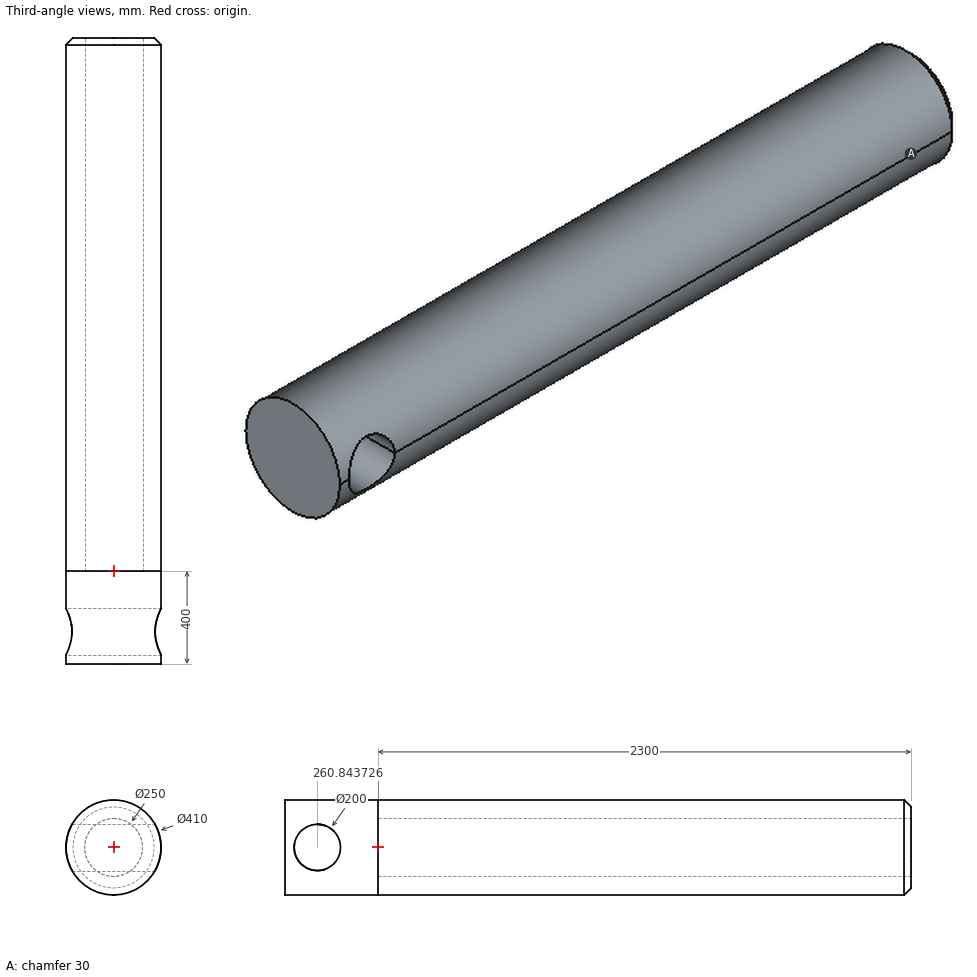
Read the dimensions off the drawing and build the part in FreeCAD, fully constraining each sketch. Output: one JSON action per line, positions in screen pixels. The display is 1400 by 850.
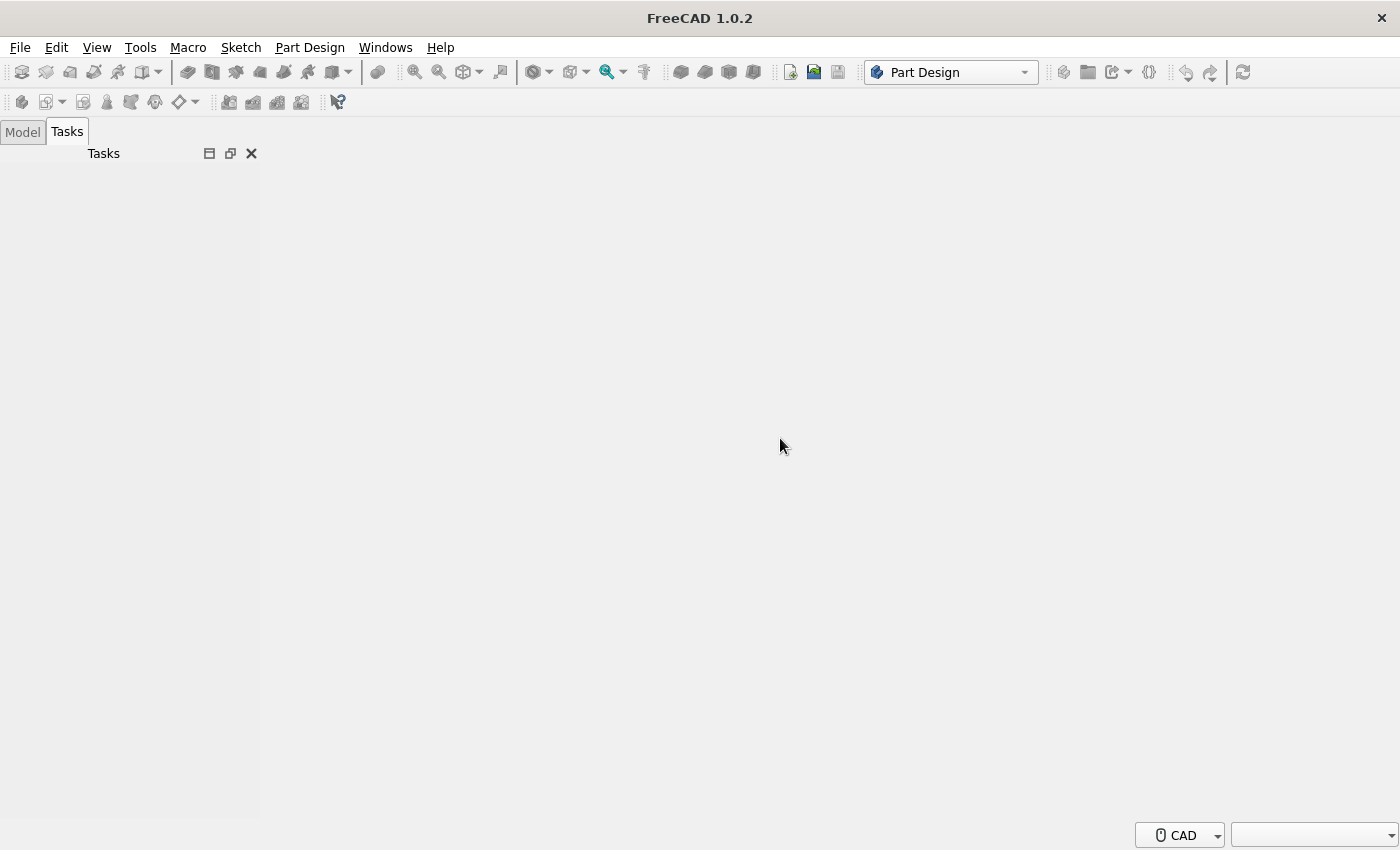
{"action": "left_click", "coordinate": [790, 72]}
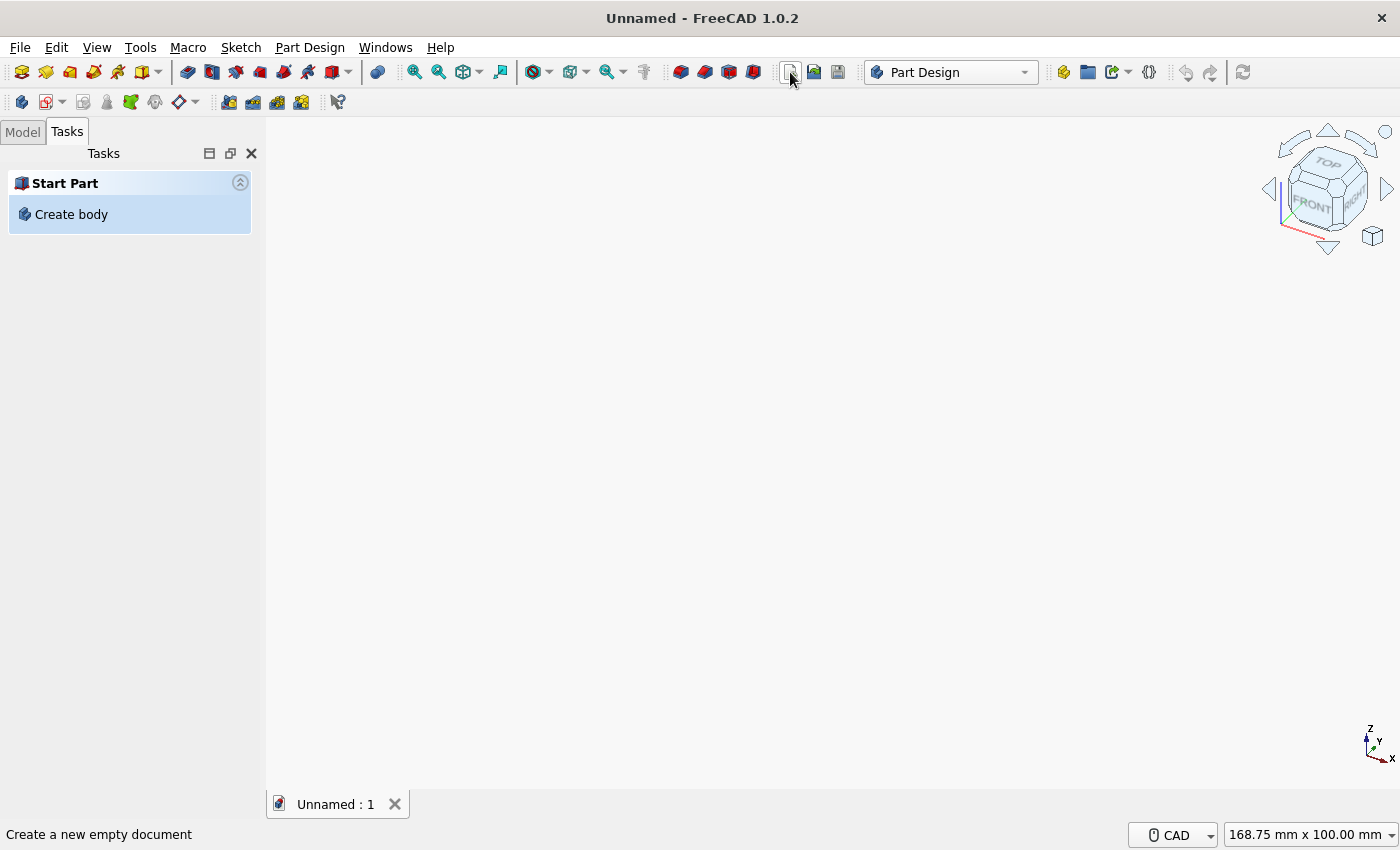
{"action": "left_click", "coordinate": [46, 102]}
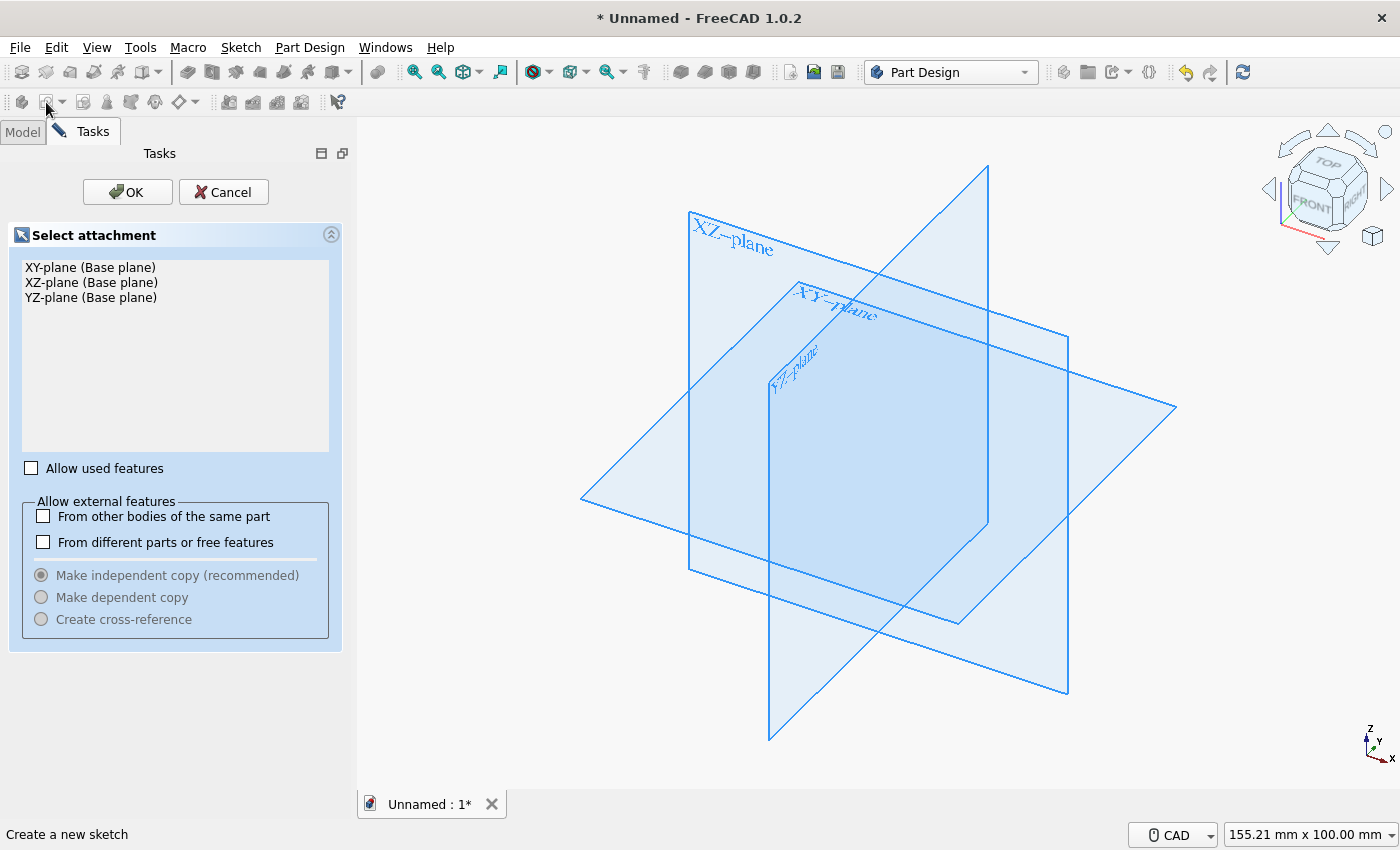
{"action": "left_click", "coordinate": [82, 282]}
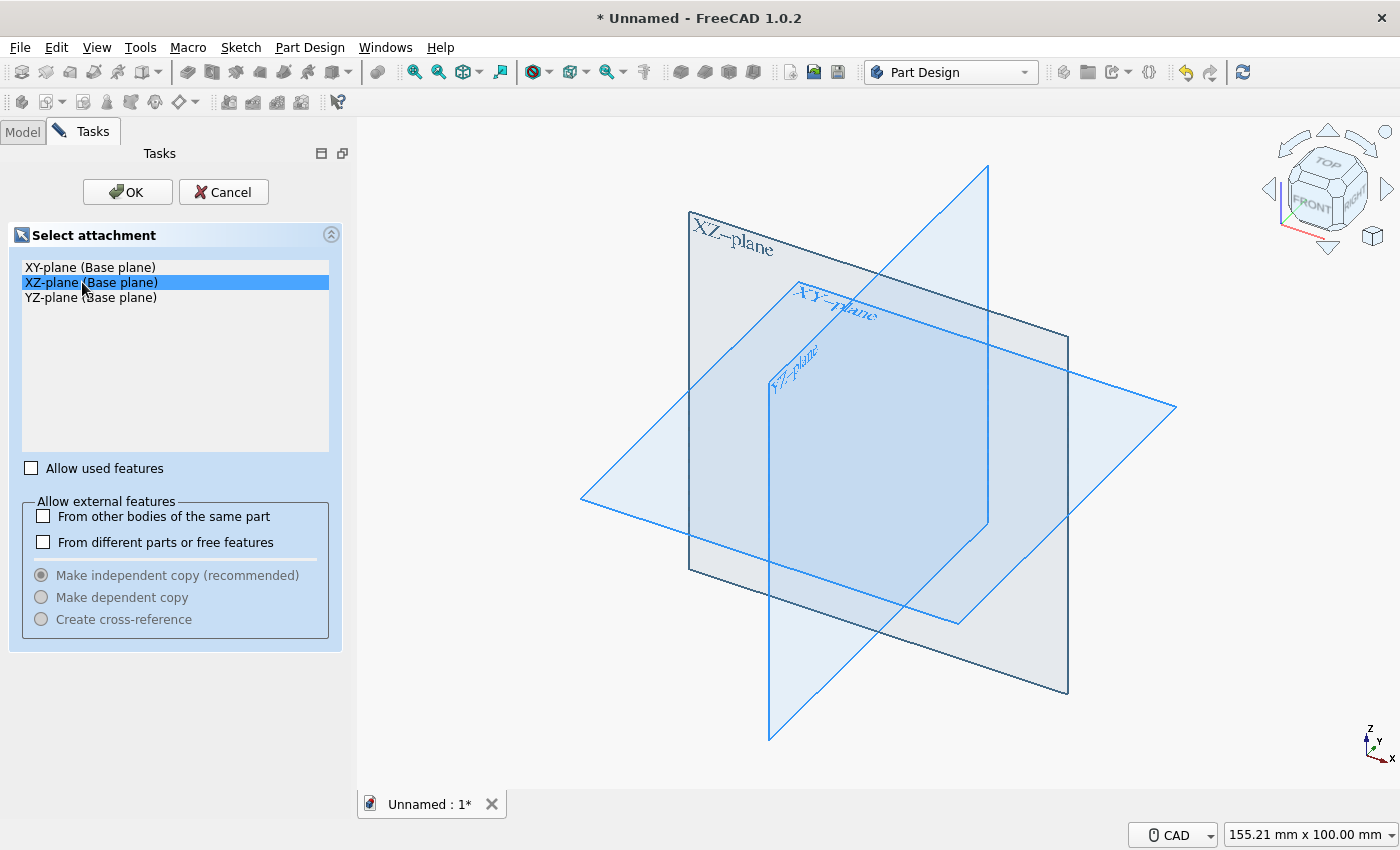
{"action": "left_click", "coordinate": [128, 192]}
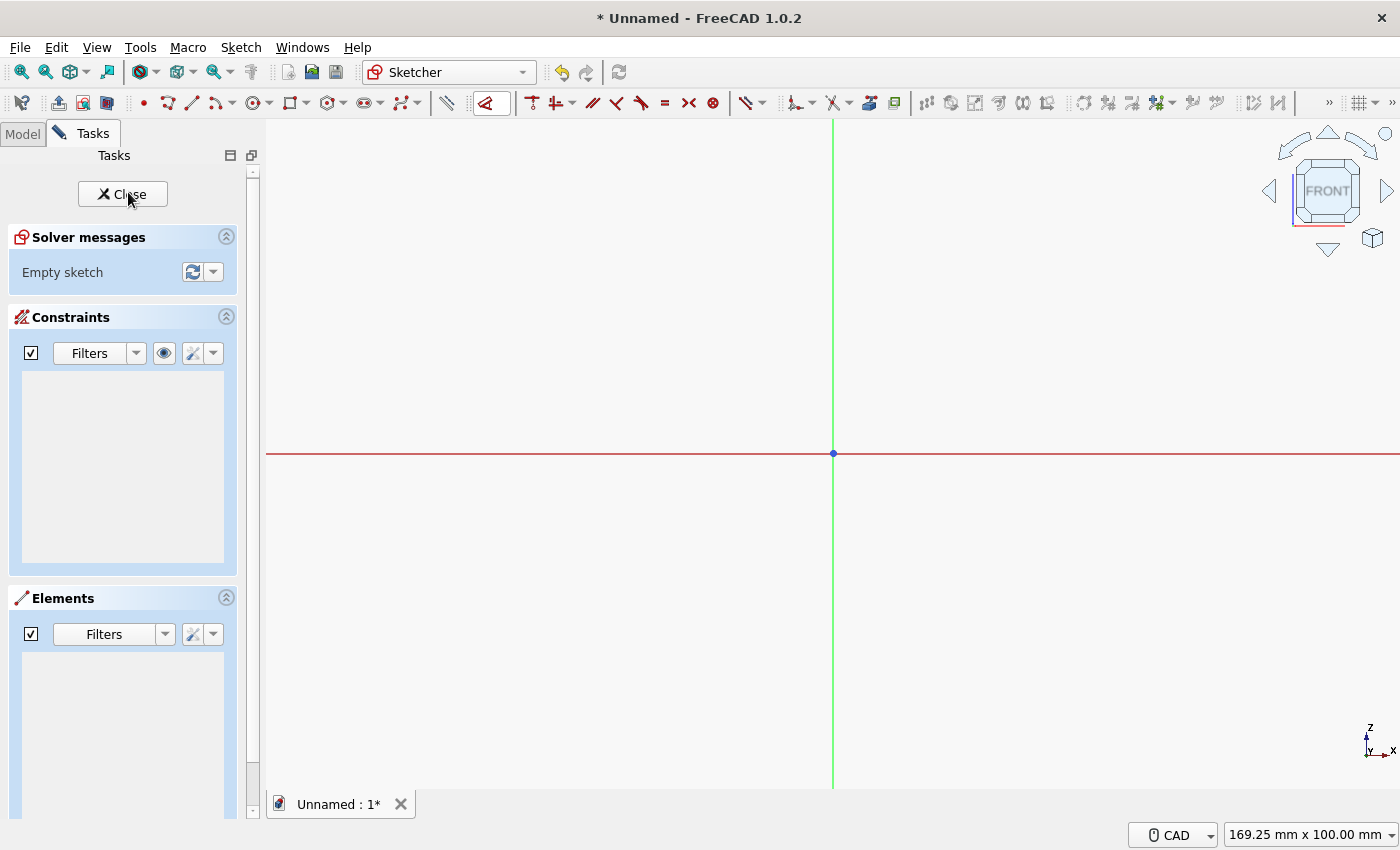
{"action": "scroll", "coordinate": [751, 454], "scroll_direction": "down", "scroll_amount": 9}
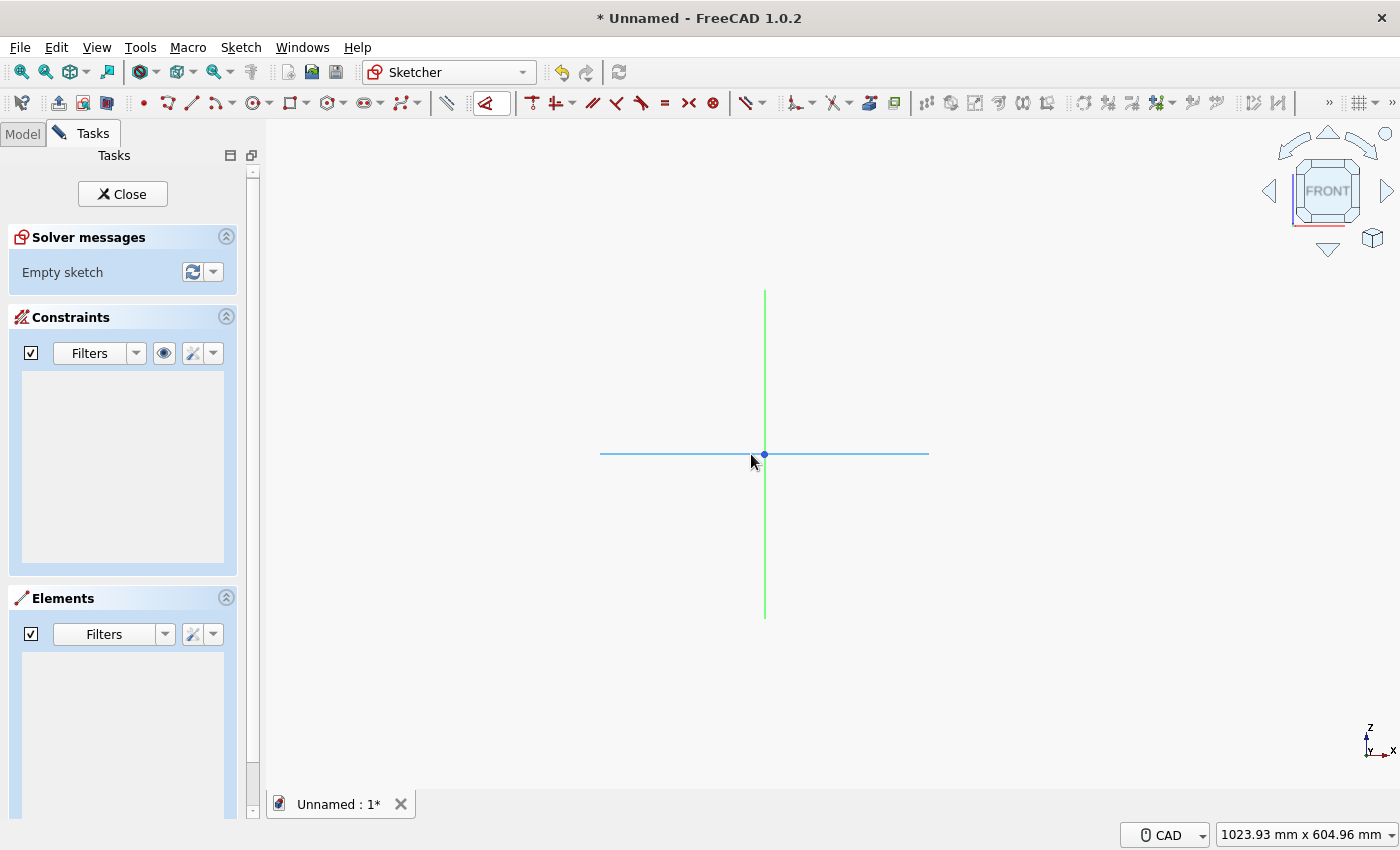
{"action": "left_click", "coordinate": [254, 104]}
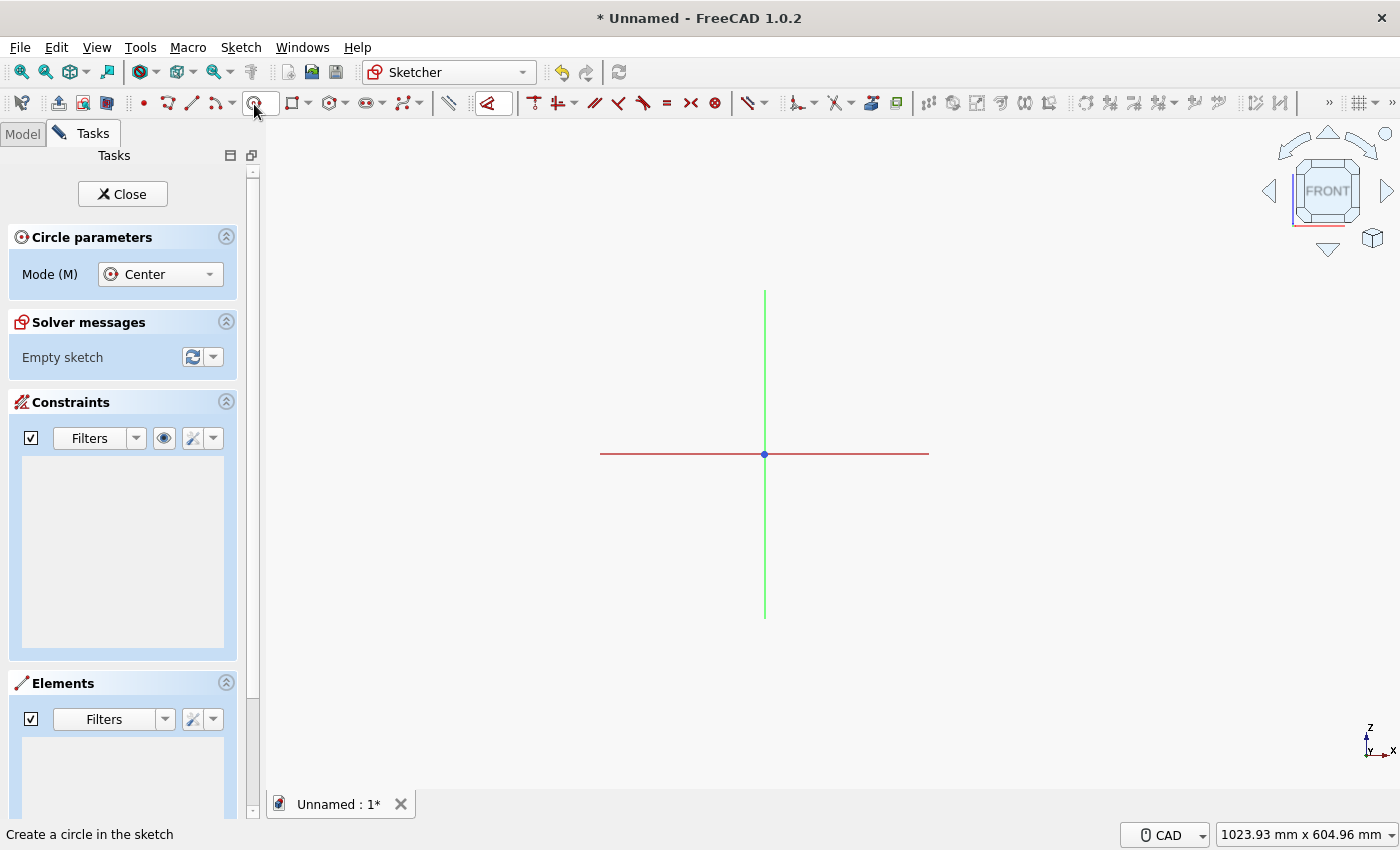
{"action": "left_click", "coordinate": [765, 454]}
{"action": "mouse_move", "coordinate": [925, 294]}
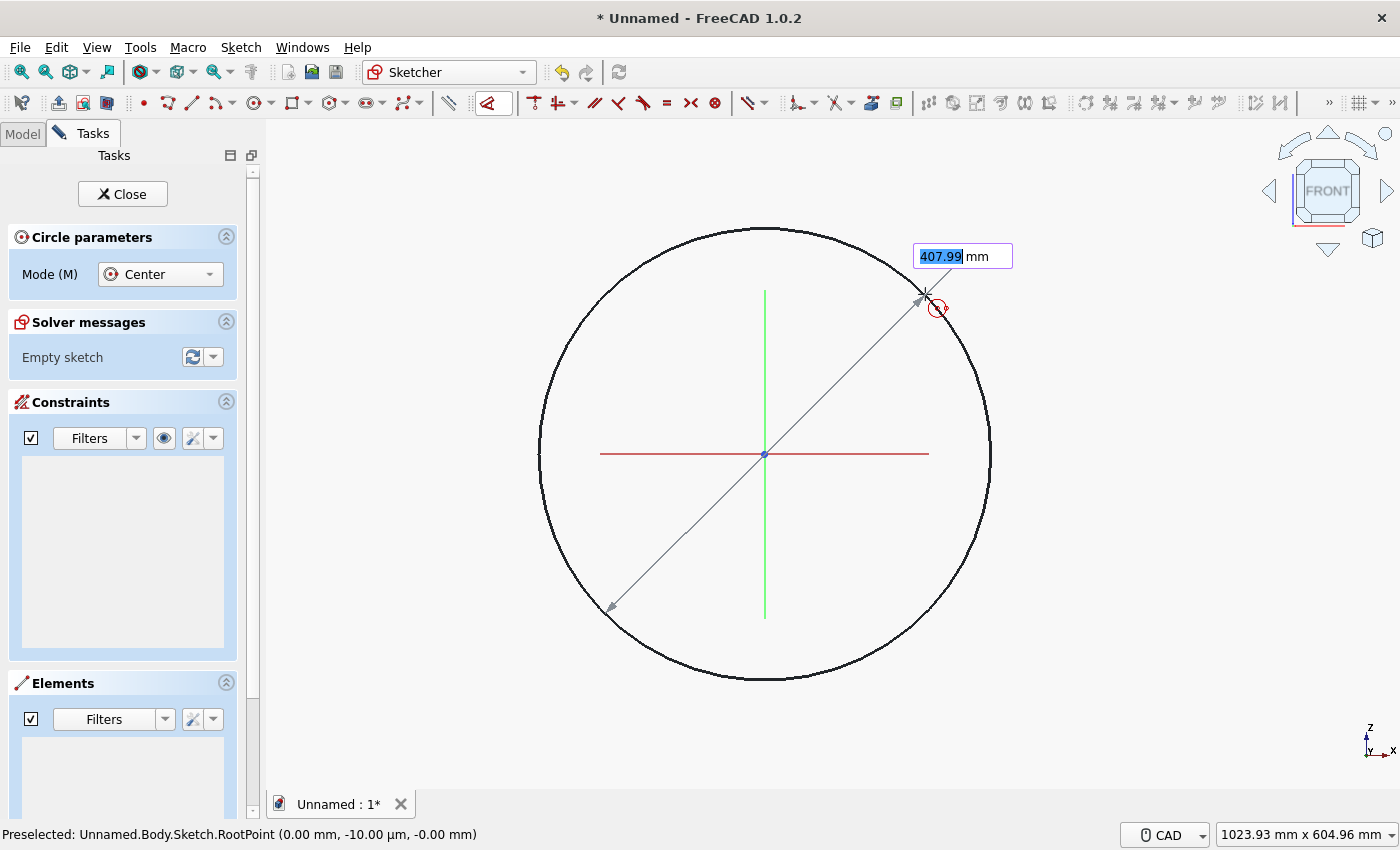
{"action": "type", "text": "410"}
{"action": "key", "text": "Return"}